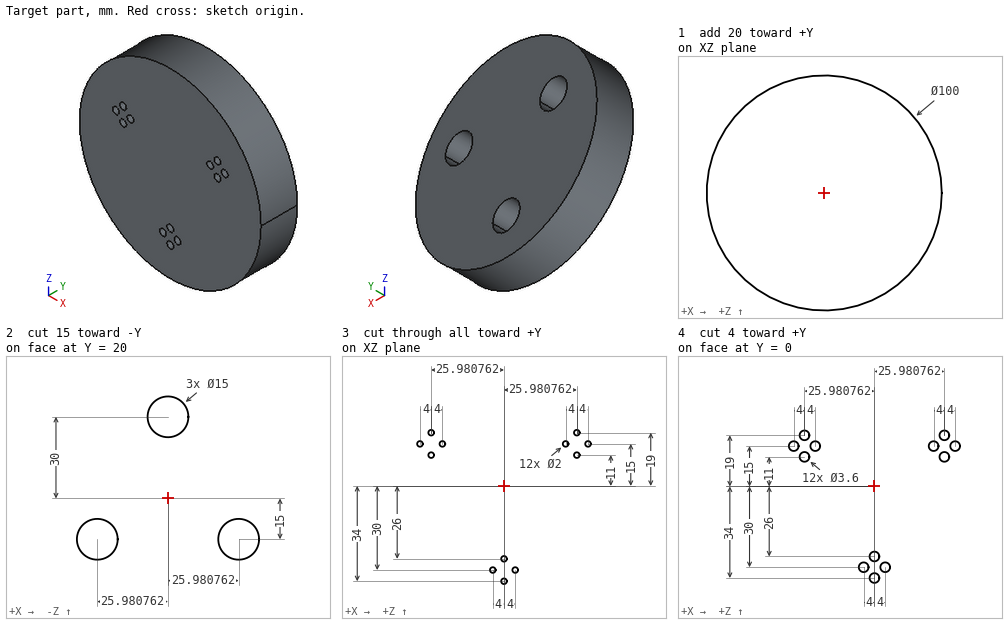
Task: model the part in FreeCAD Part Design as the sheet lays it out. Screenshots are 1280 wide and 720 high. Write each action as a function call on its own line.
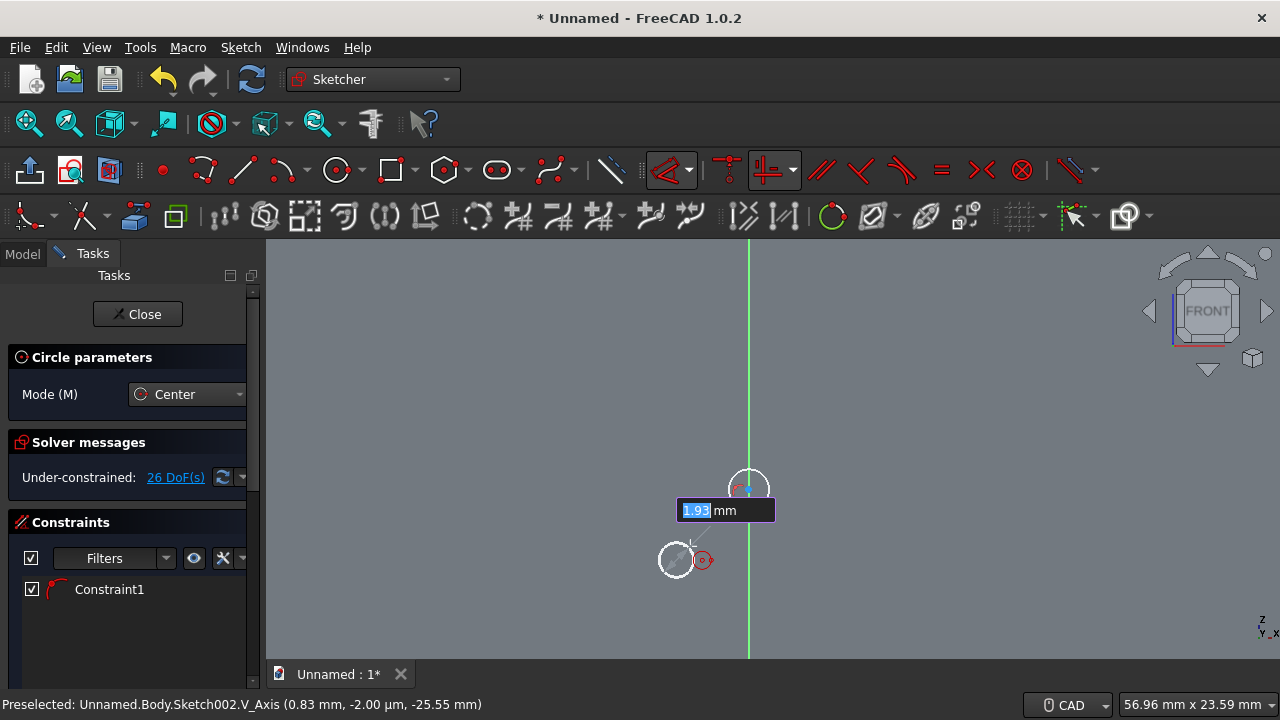
click(690, 542)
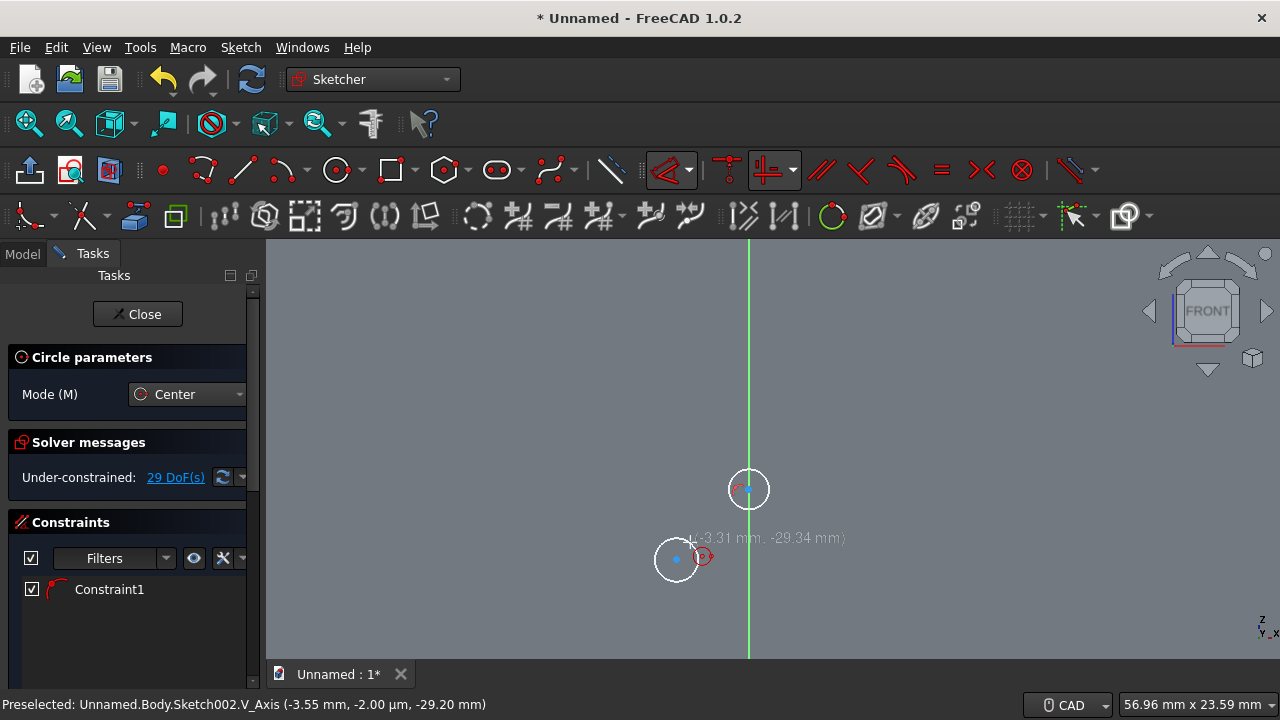
scroll(749, 626, up, 2)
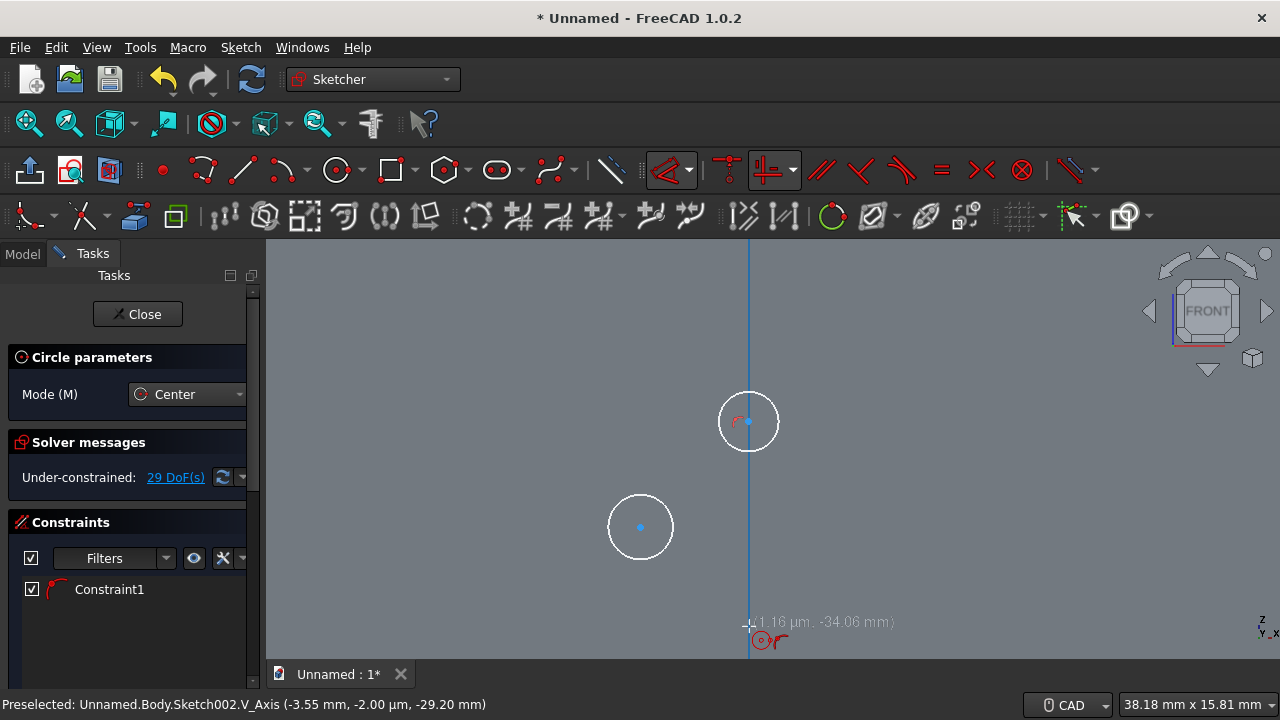
scroll(696, 553, down, 9)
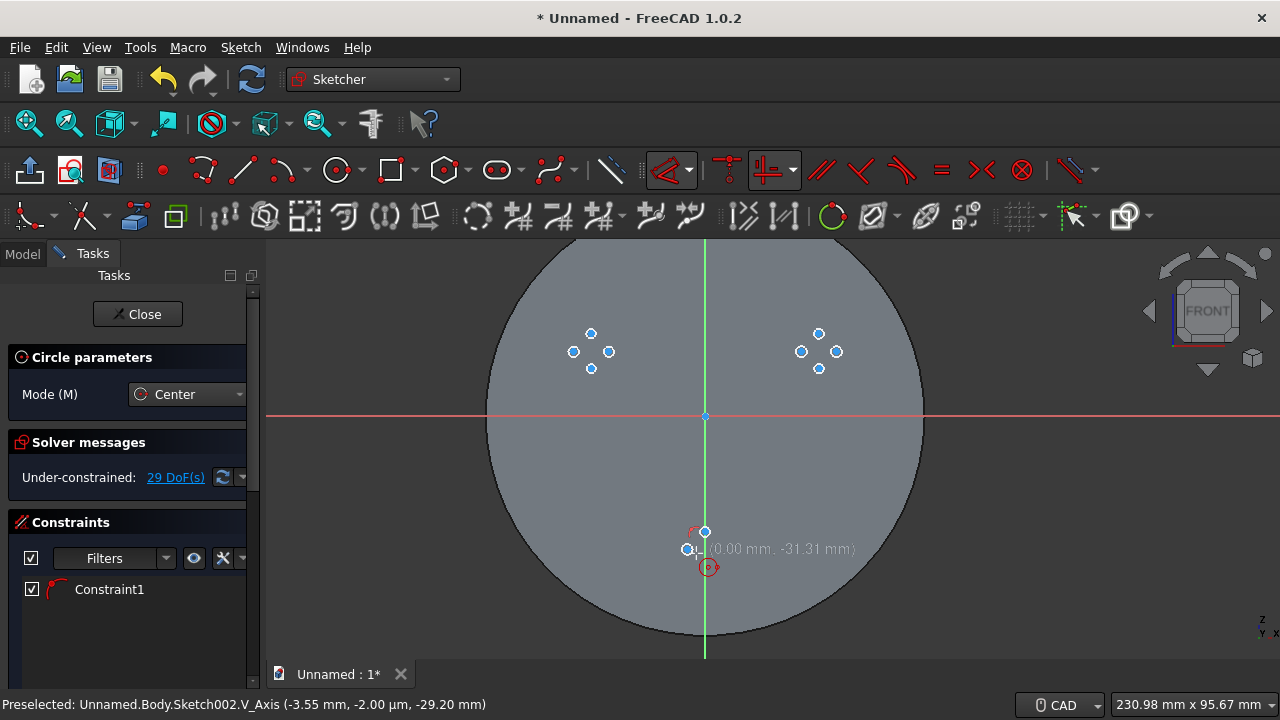
click(705, 566)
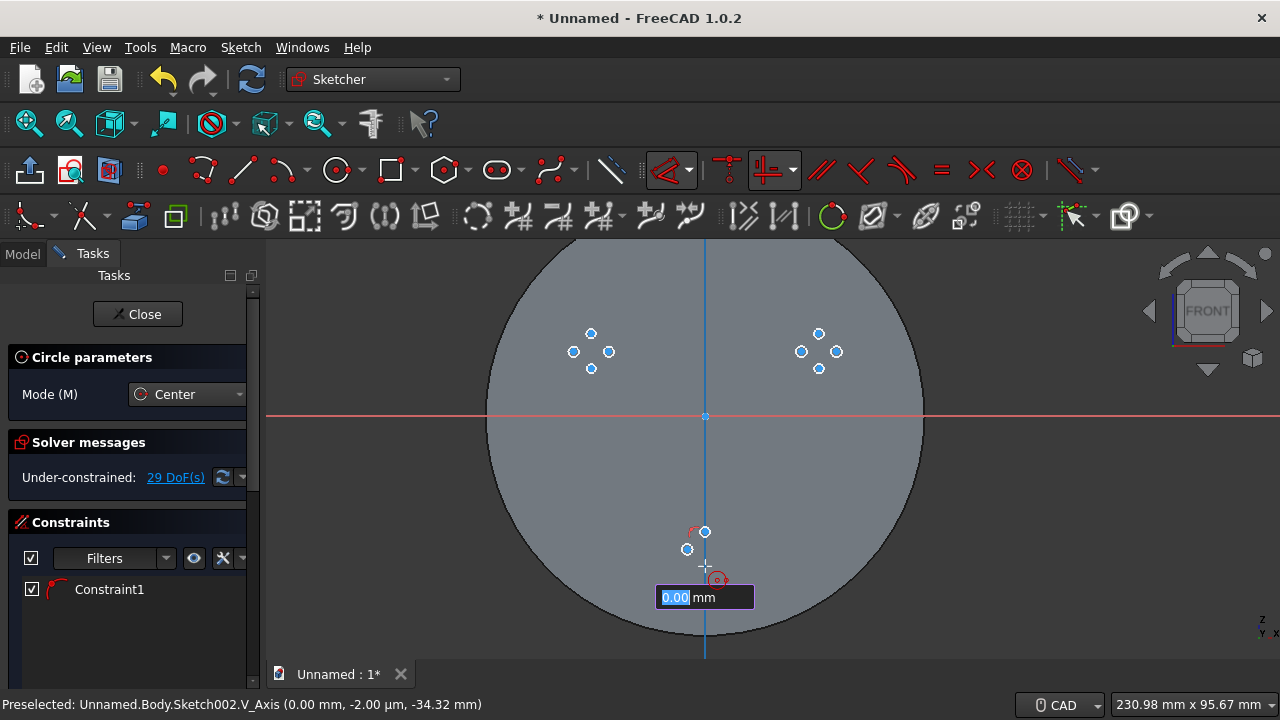
scroll(709, 564, up, 7)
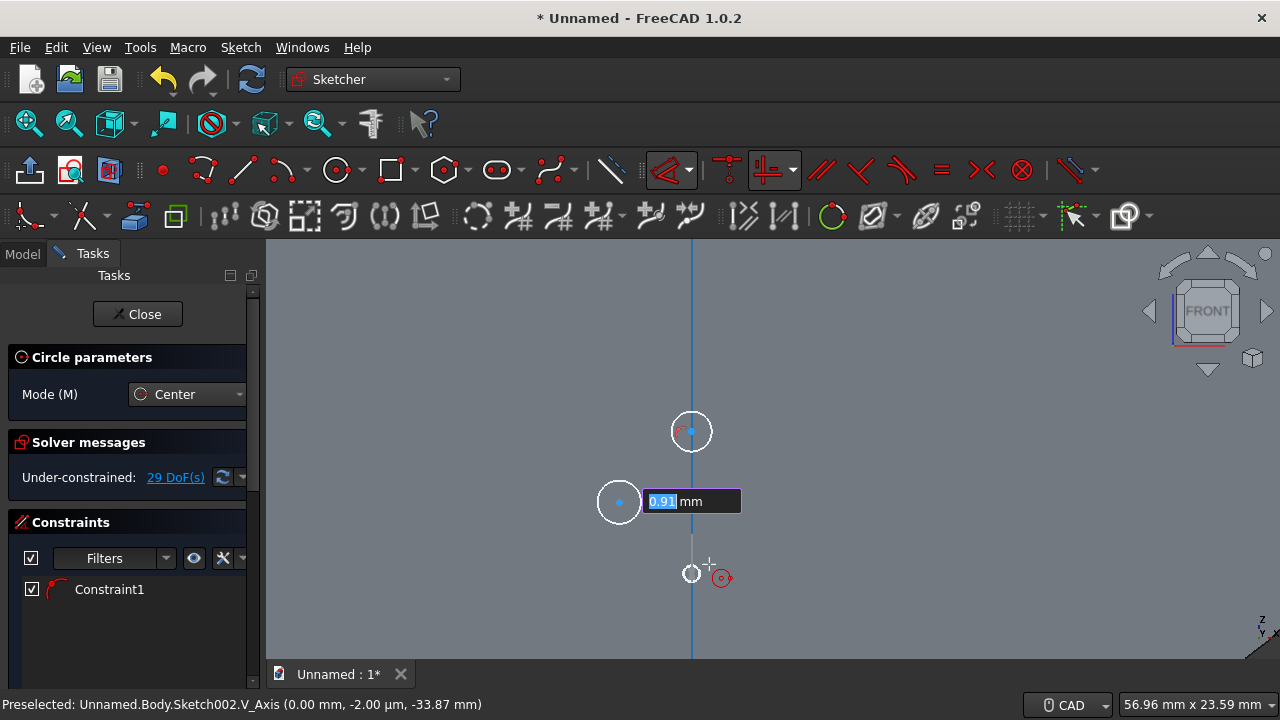
click(708, 562)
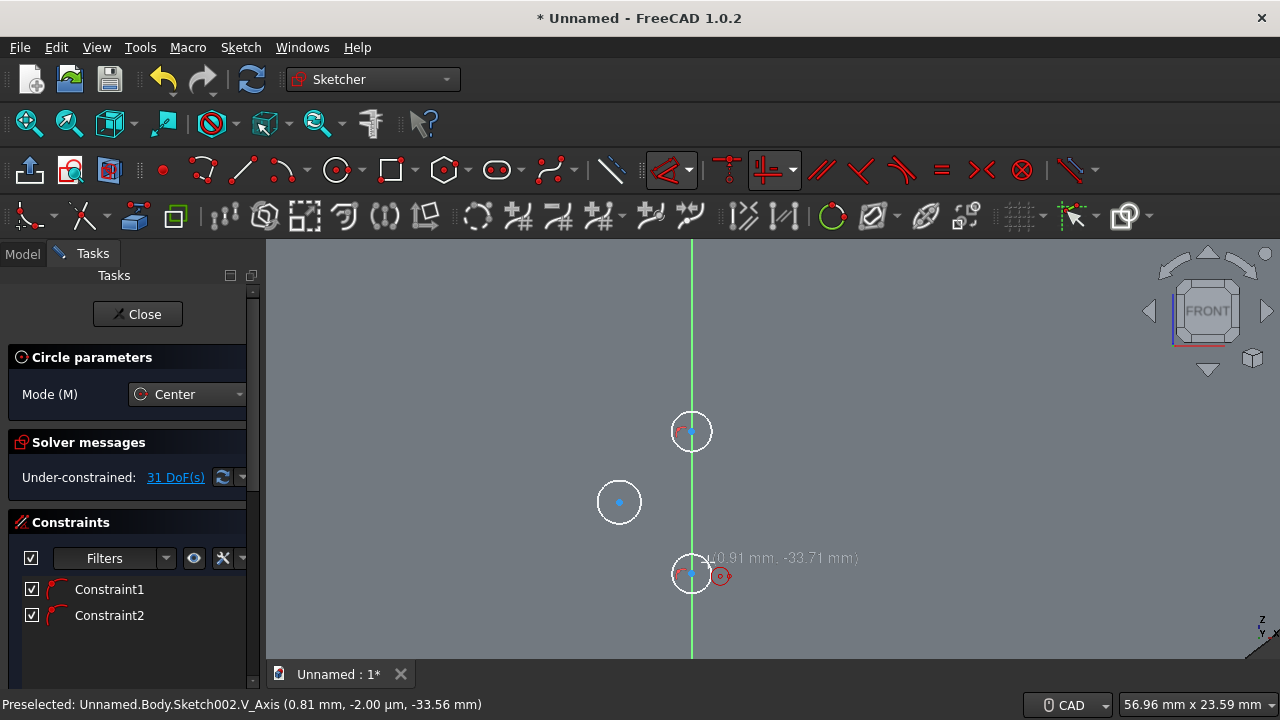
scroll(763, 497, up, 2)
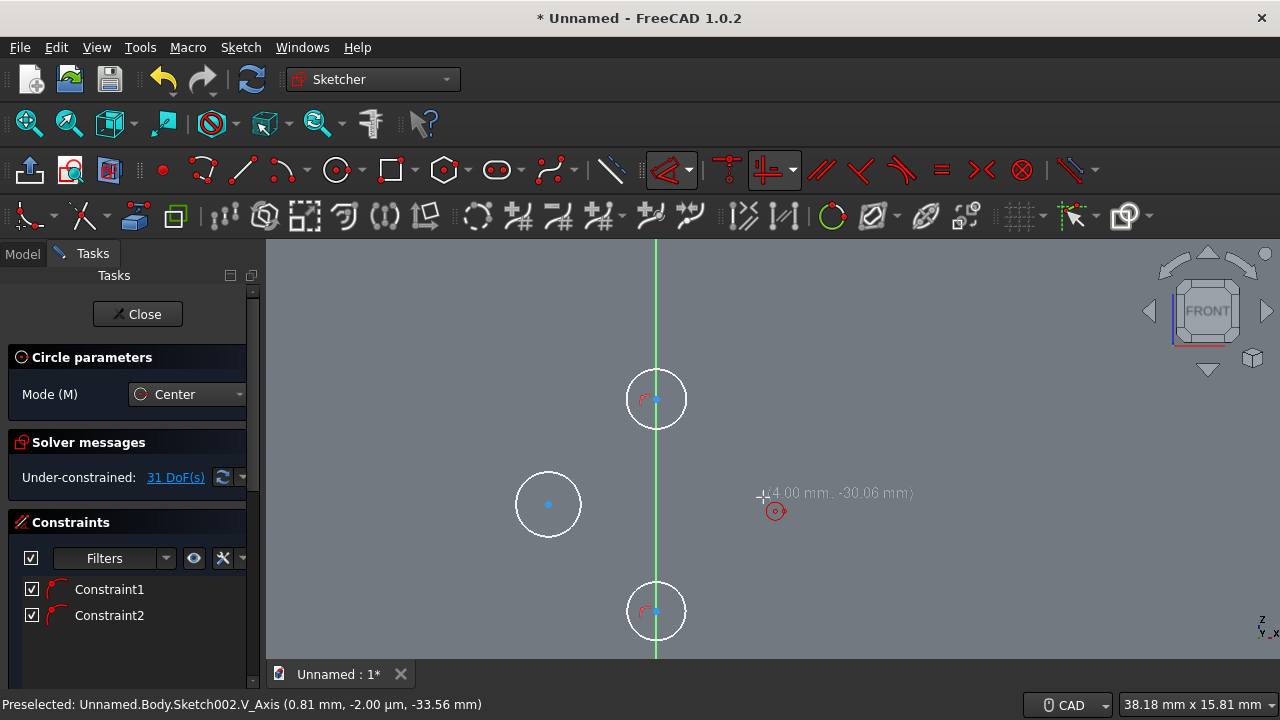
scroll(714, 558, down, 9)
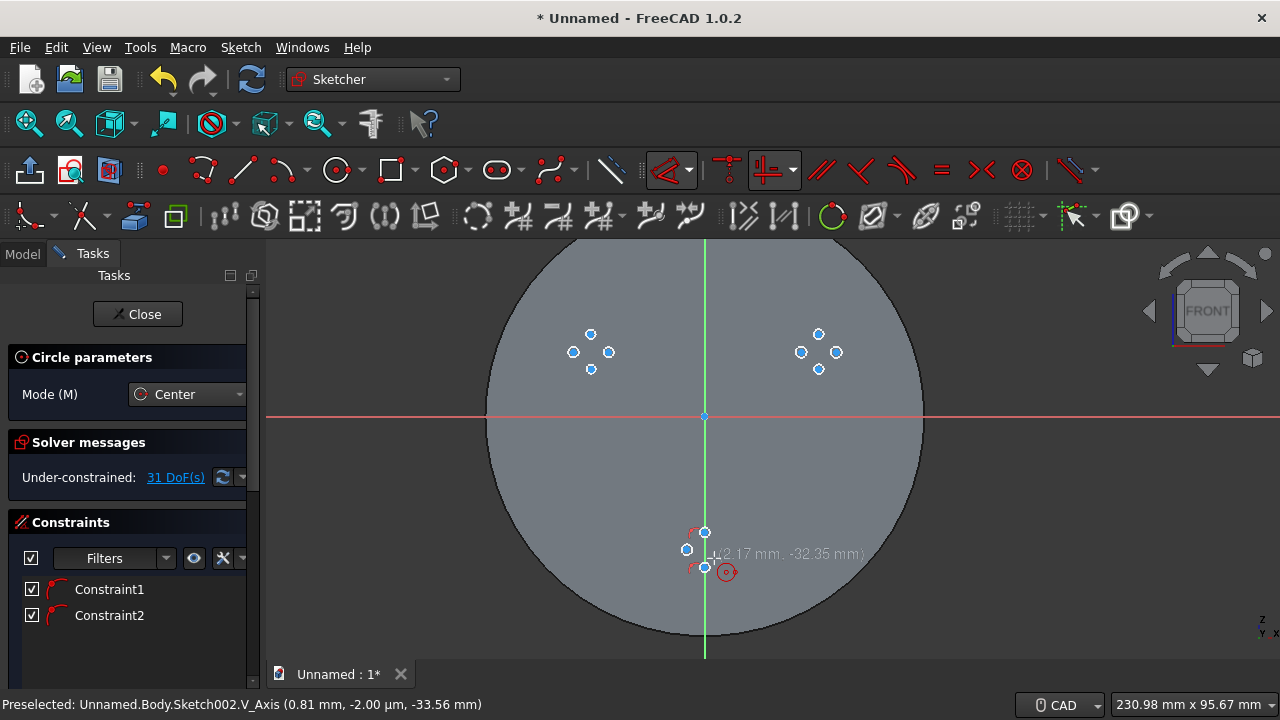
click(722, 548)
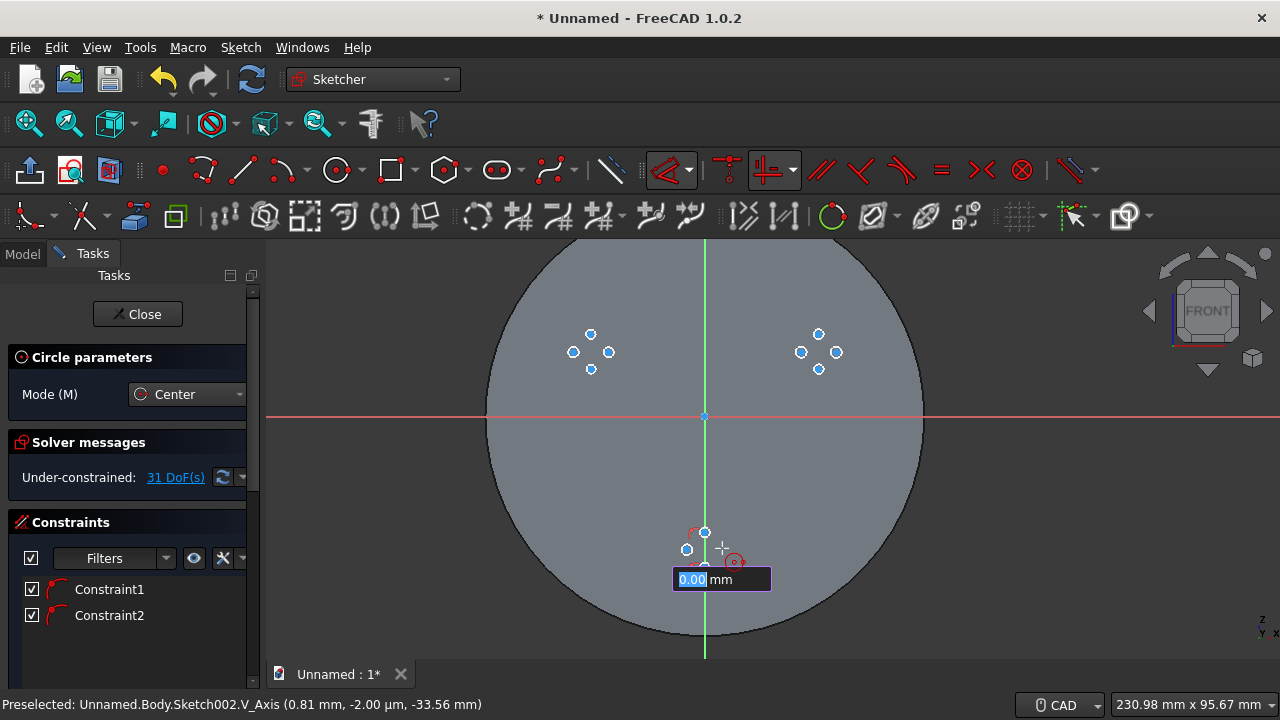
scroll(726, 545, up, 7)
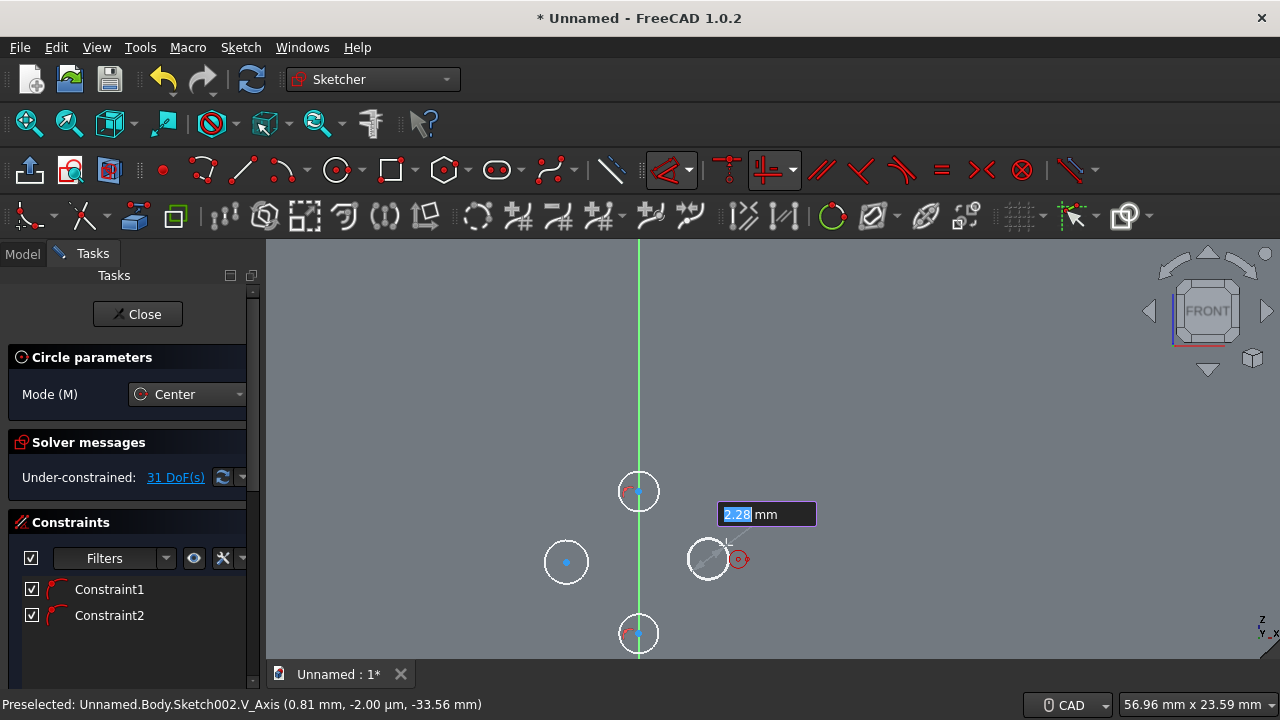
click(723, 544)
key(Escape)